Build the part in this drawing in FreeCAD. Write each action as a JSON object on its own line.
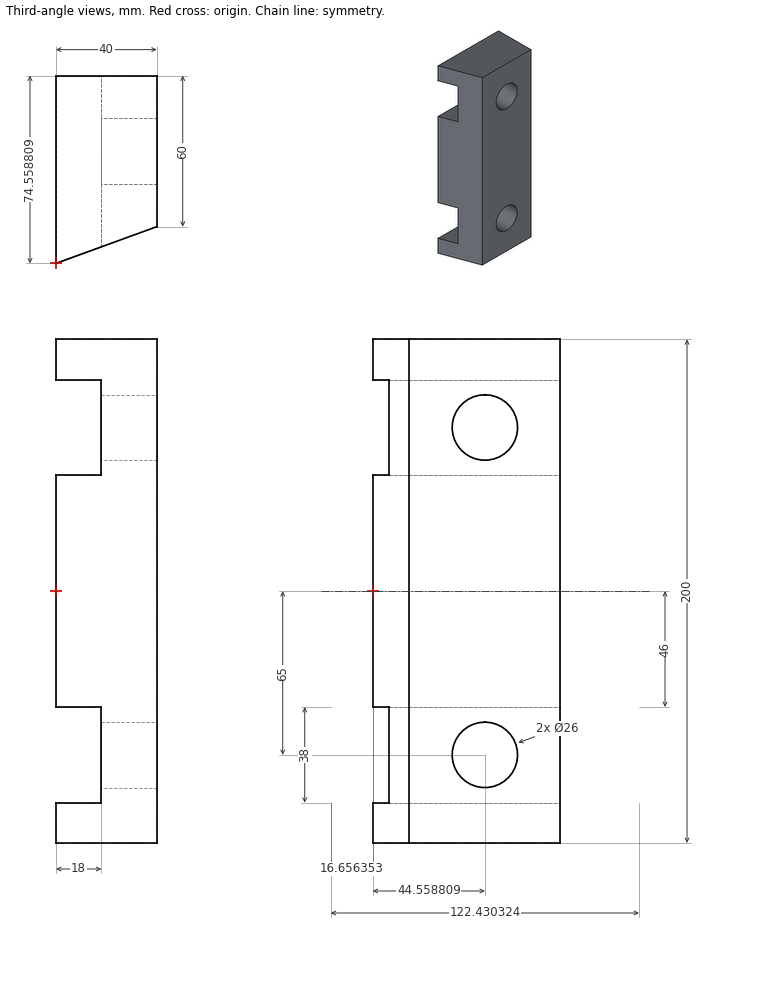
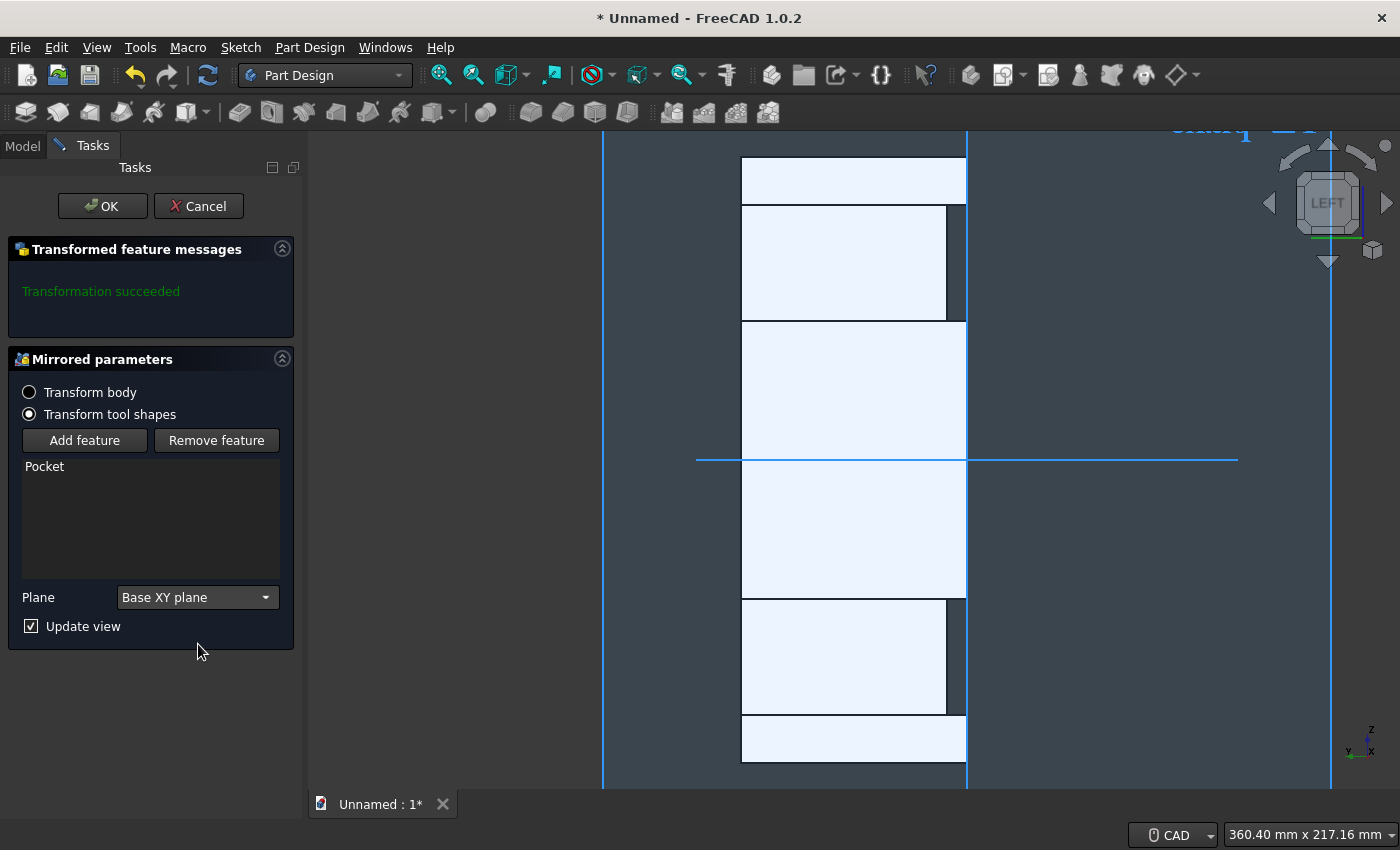
{"action": "left_click", "coordinate": [103, 206]}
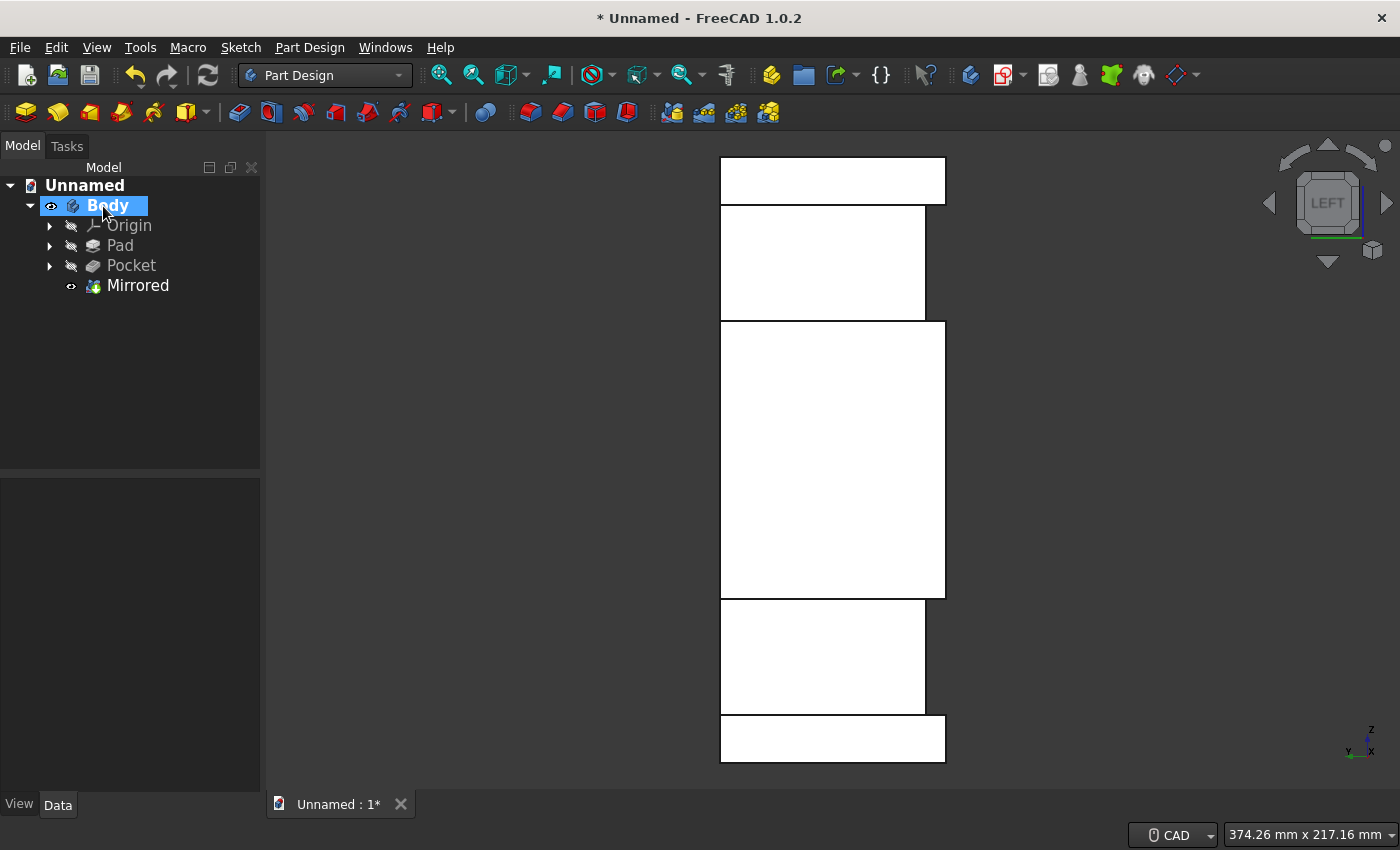
{"action": "left_click", "coordinate": [833, 459]}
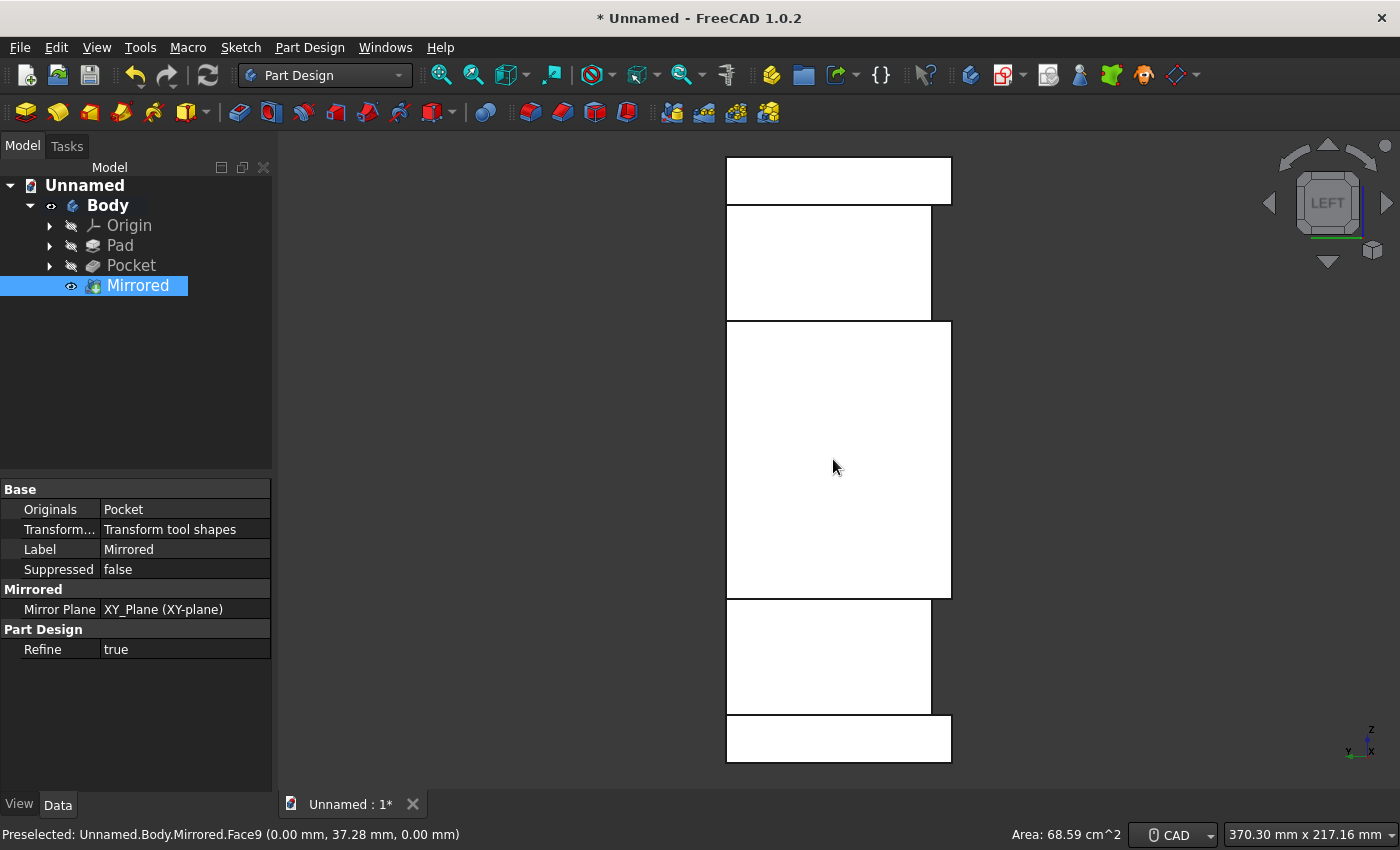
{"action": "left_click", "coordinate": [1004, 76]}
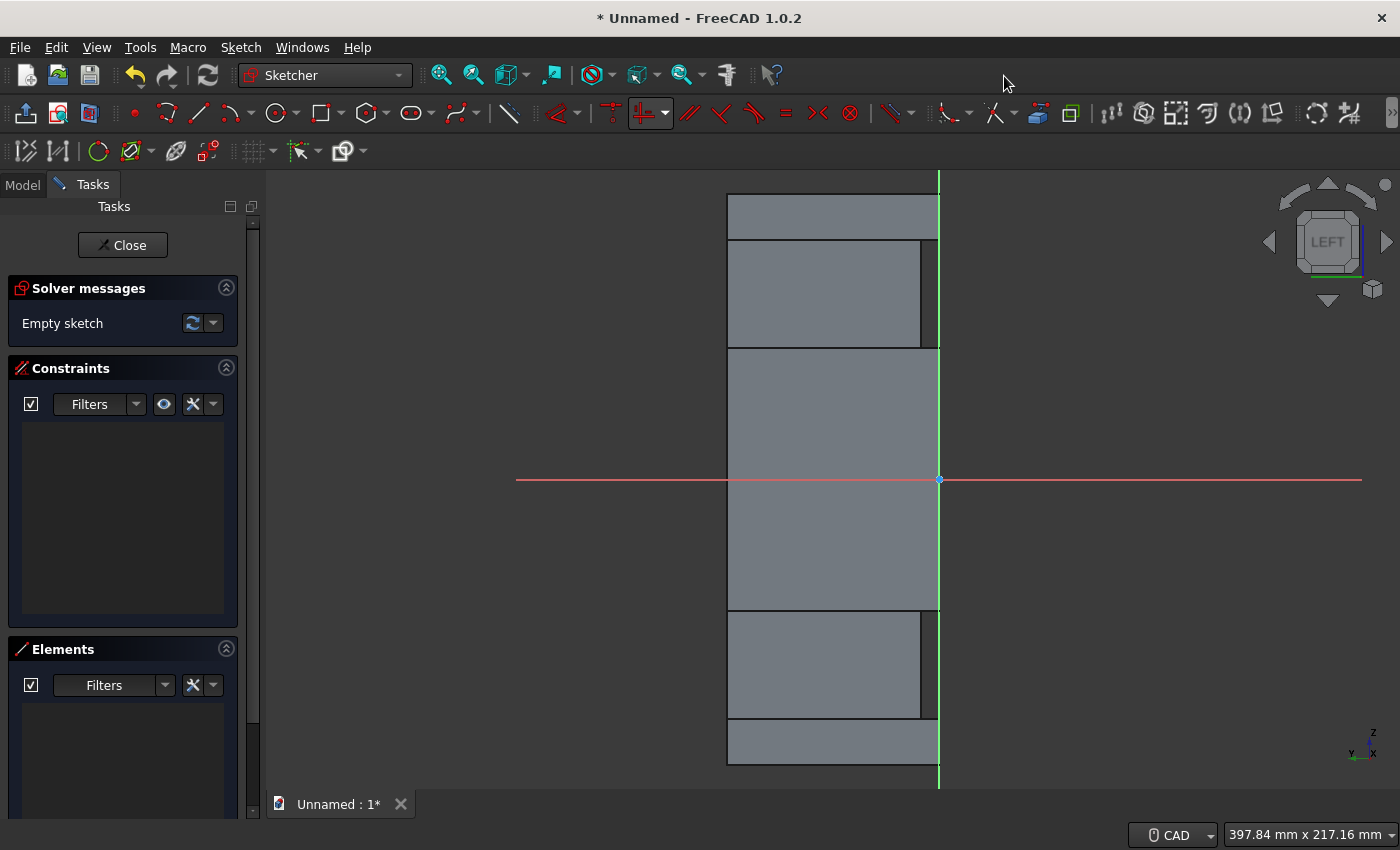
{"action": "left_click", "coordinate": [276, 114]}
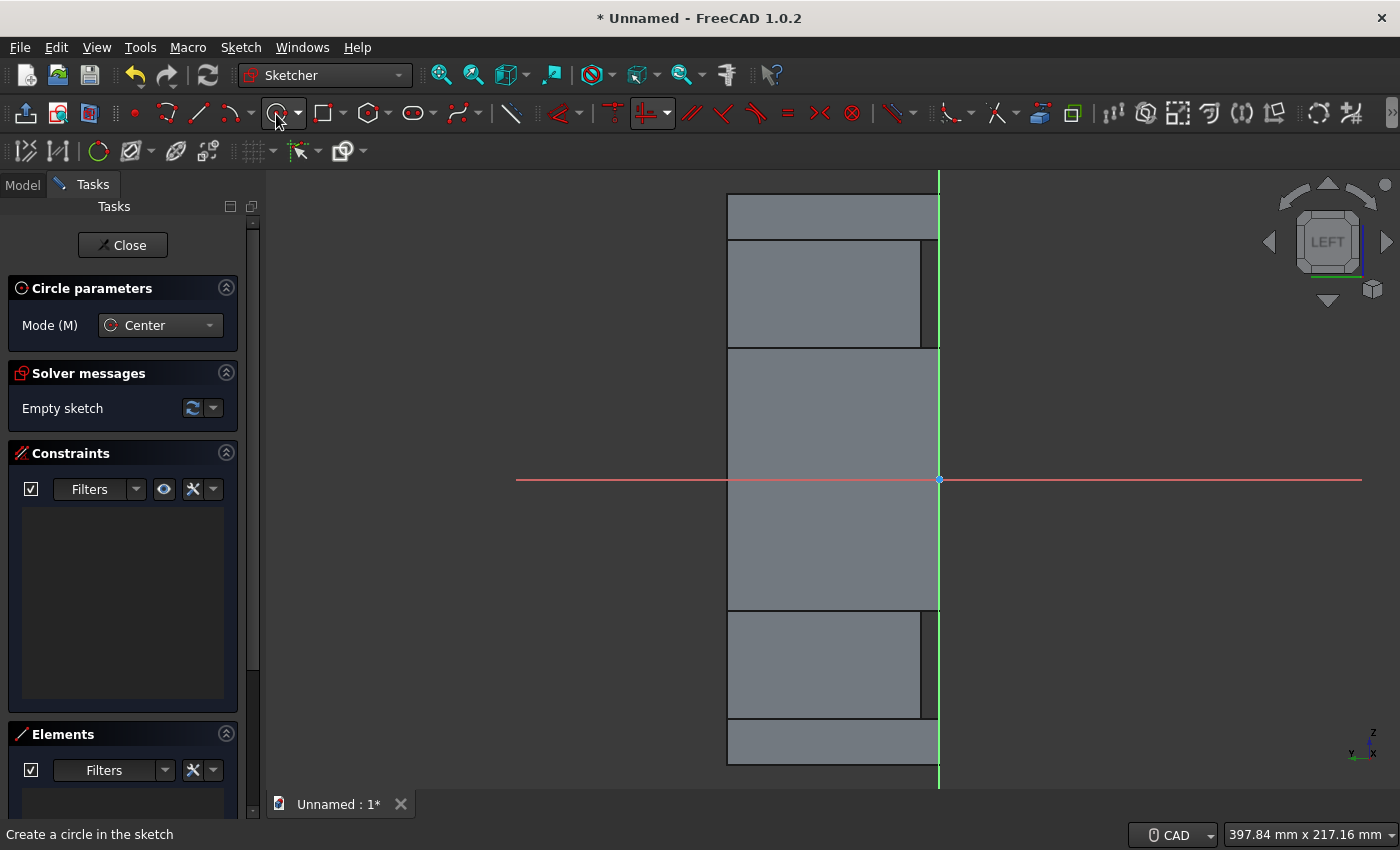
{"action": "left_click", "coordinate": [812, 665]}
{"action": "mouse_move", "coordinate": [838, 639]}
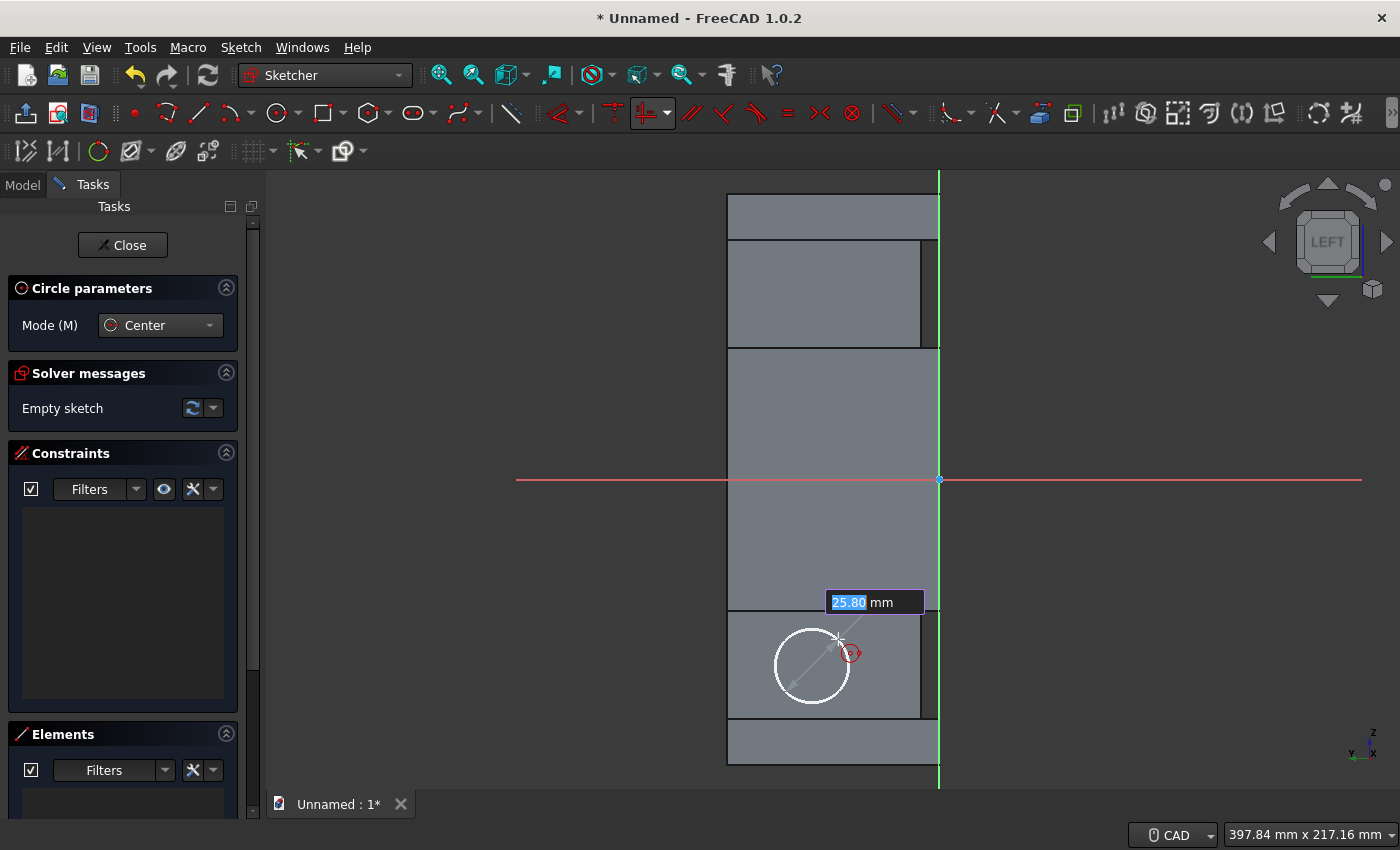
{"action": "type", "text": "26"}
{"action": "key", "text": "Return"}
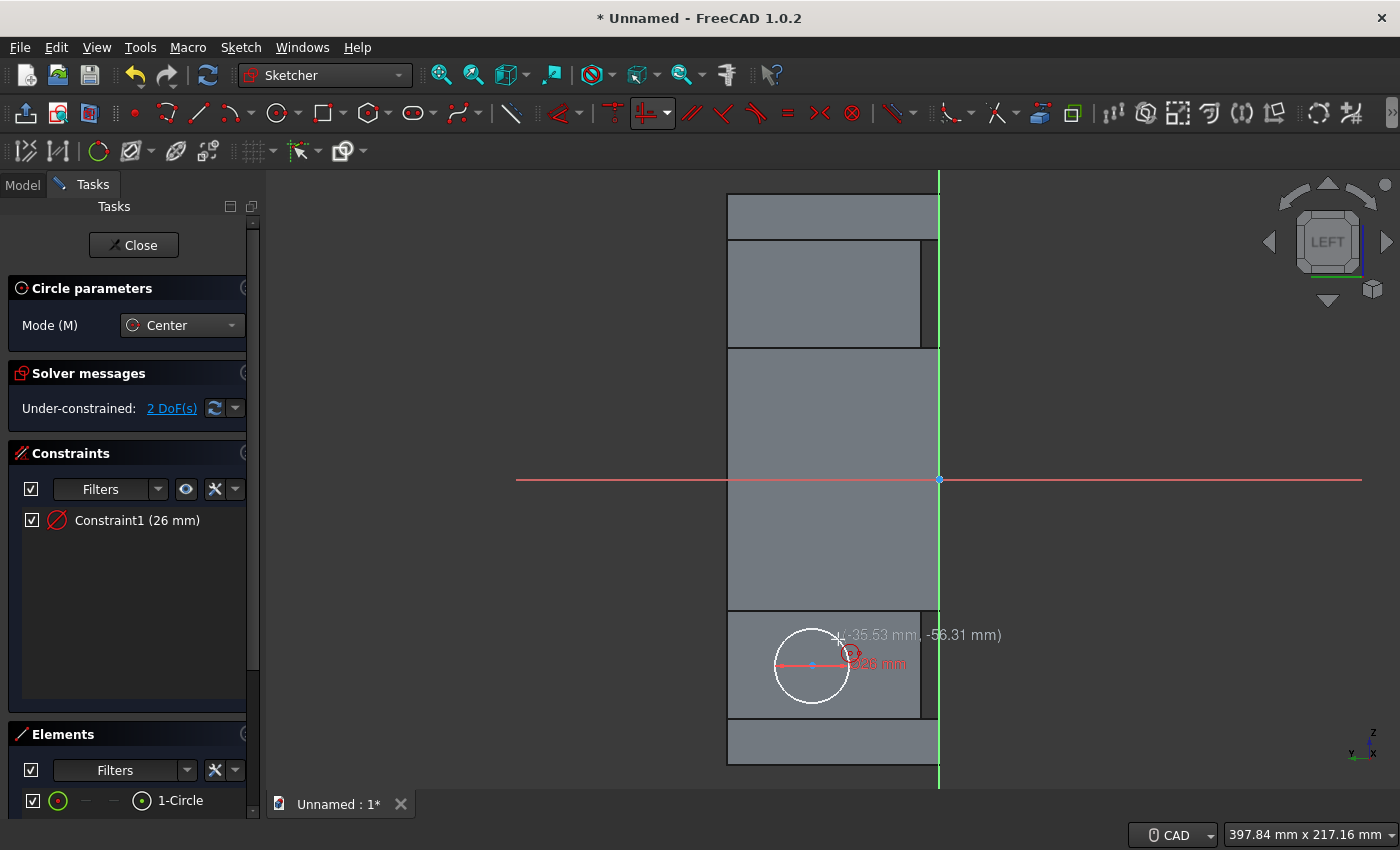
{"action": "left_click", "coordinate": [812, 294]}
{"action": "mouse_move", "coordinate": [838, 268]}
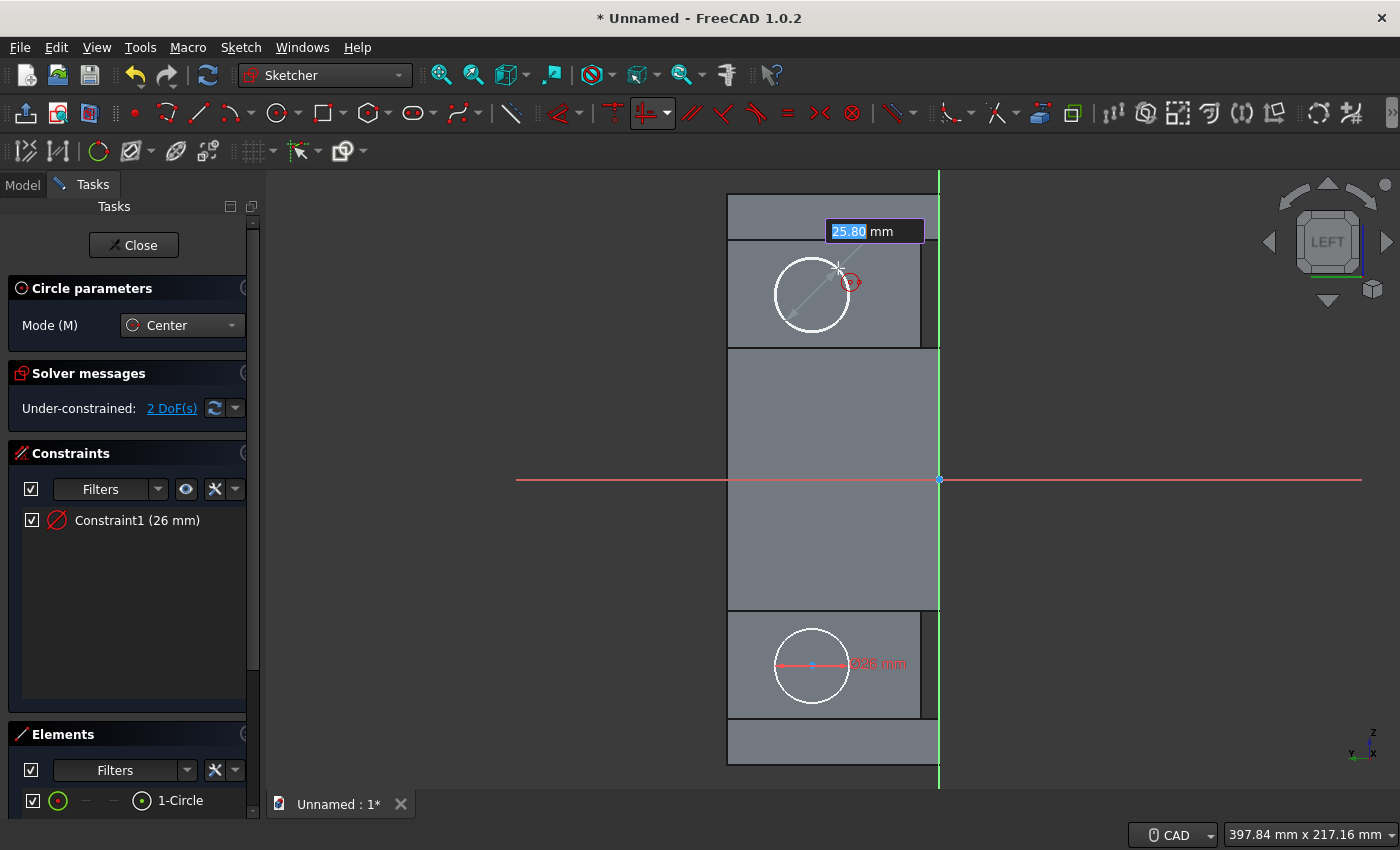
{"action": "type", "text": "26"}
{"action": "key", "text": "Return"}
{"action": "key", "text": "Escape"}